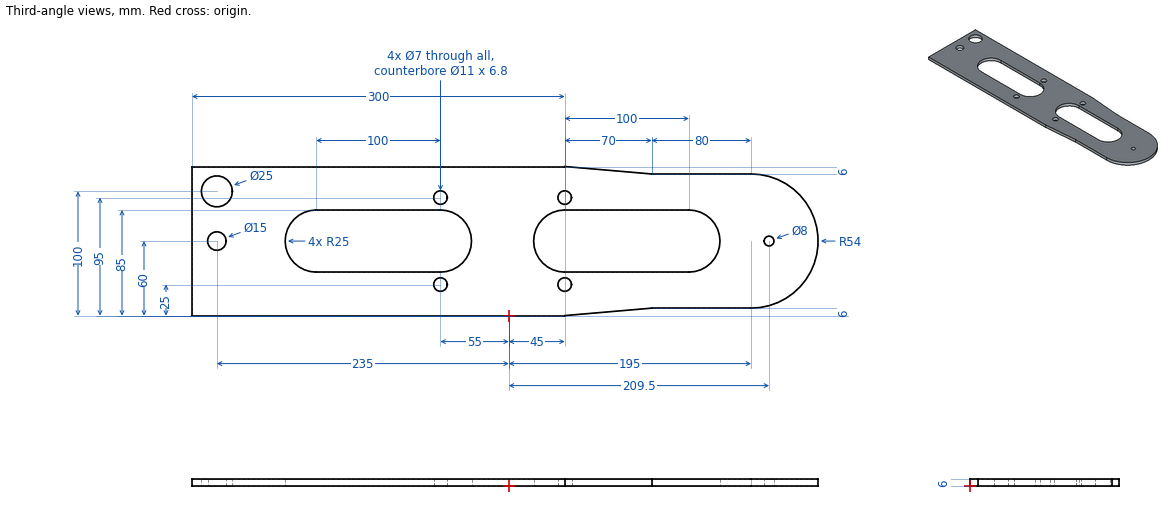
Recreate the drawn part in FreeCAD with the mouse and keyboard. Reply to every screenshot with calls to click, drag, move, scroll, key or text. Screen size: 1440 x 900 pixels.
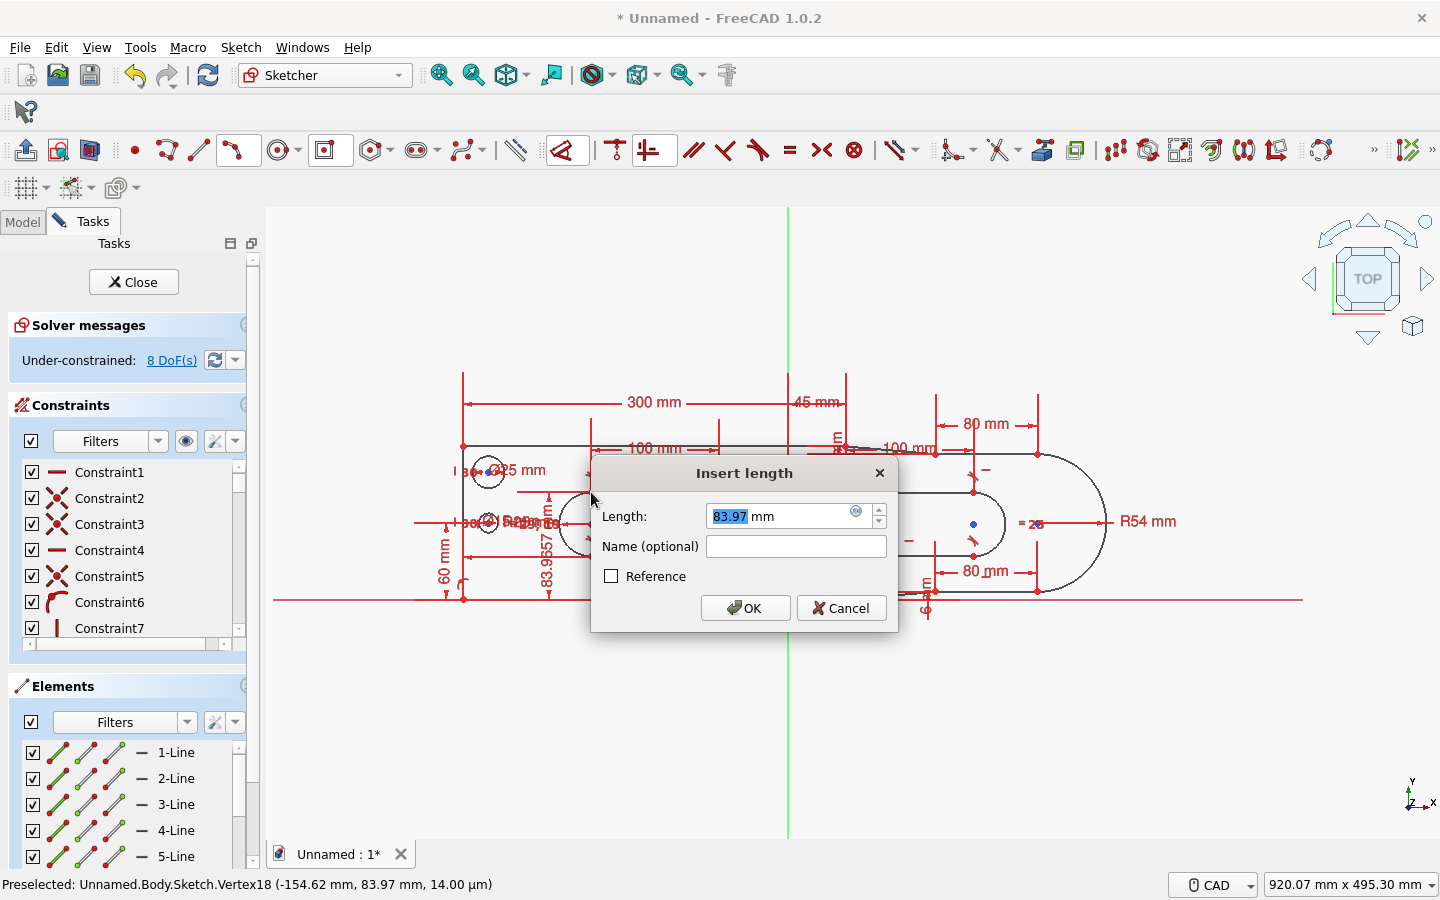
text(85)
key(Return)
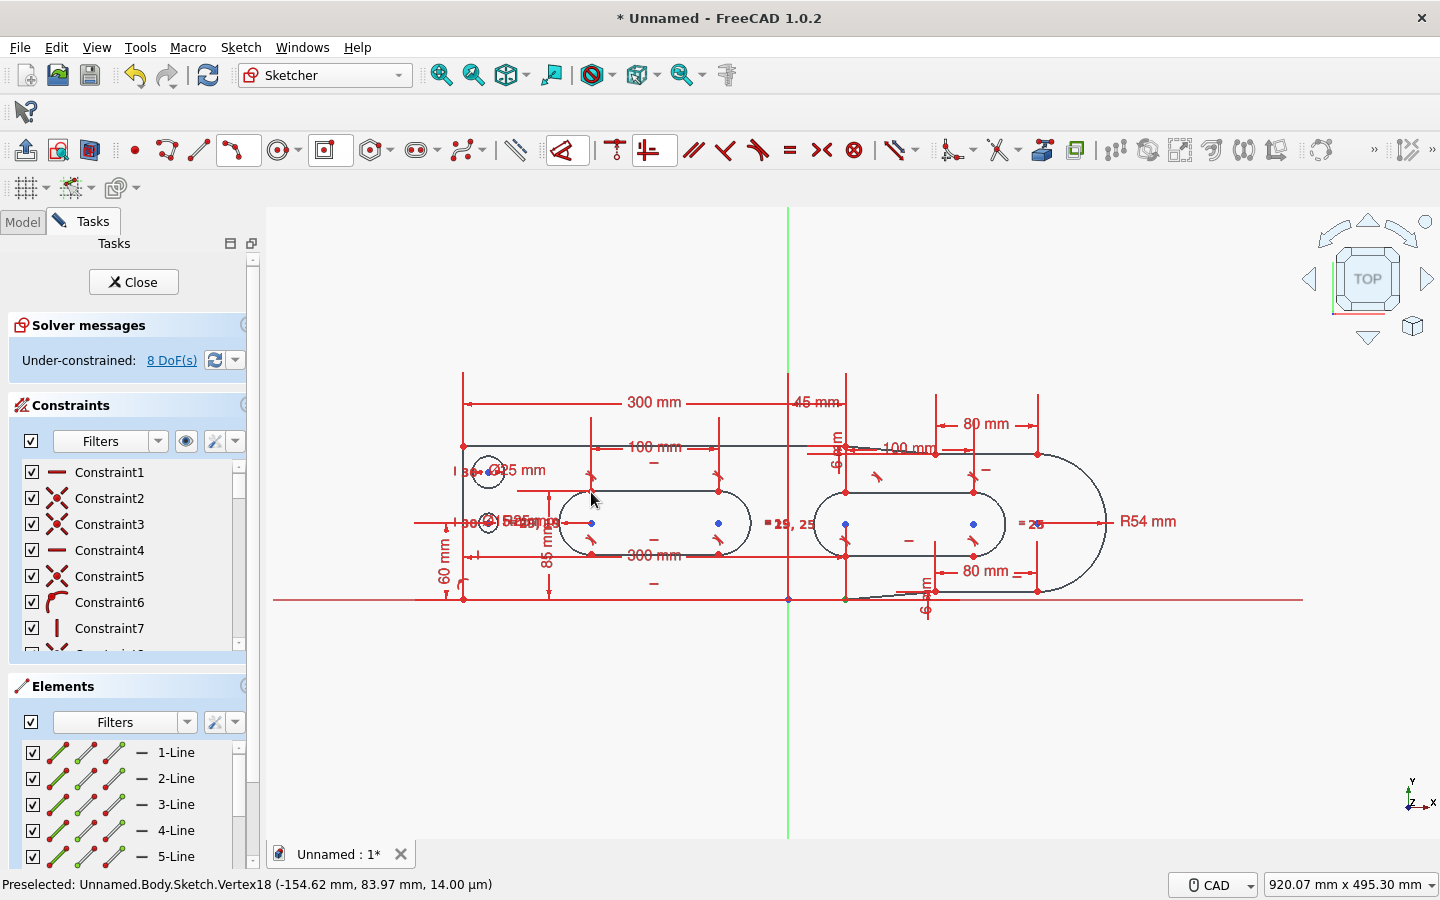
click(719, 555)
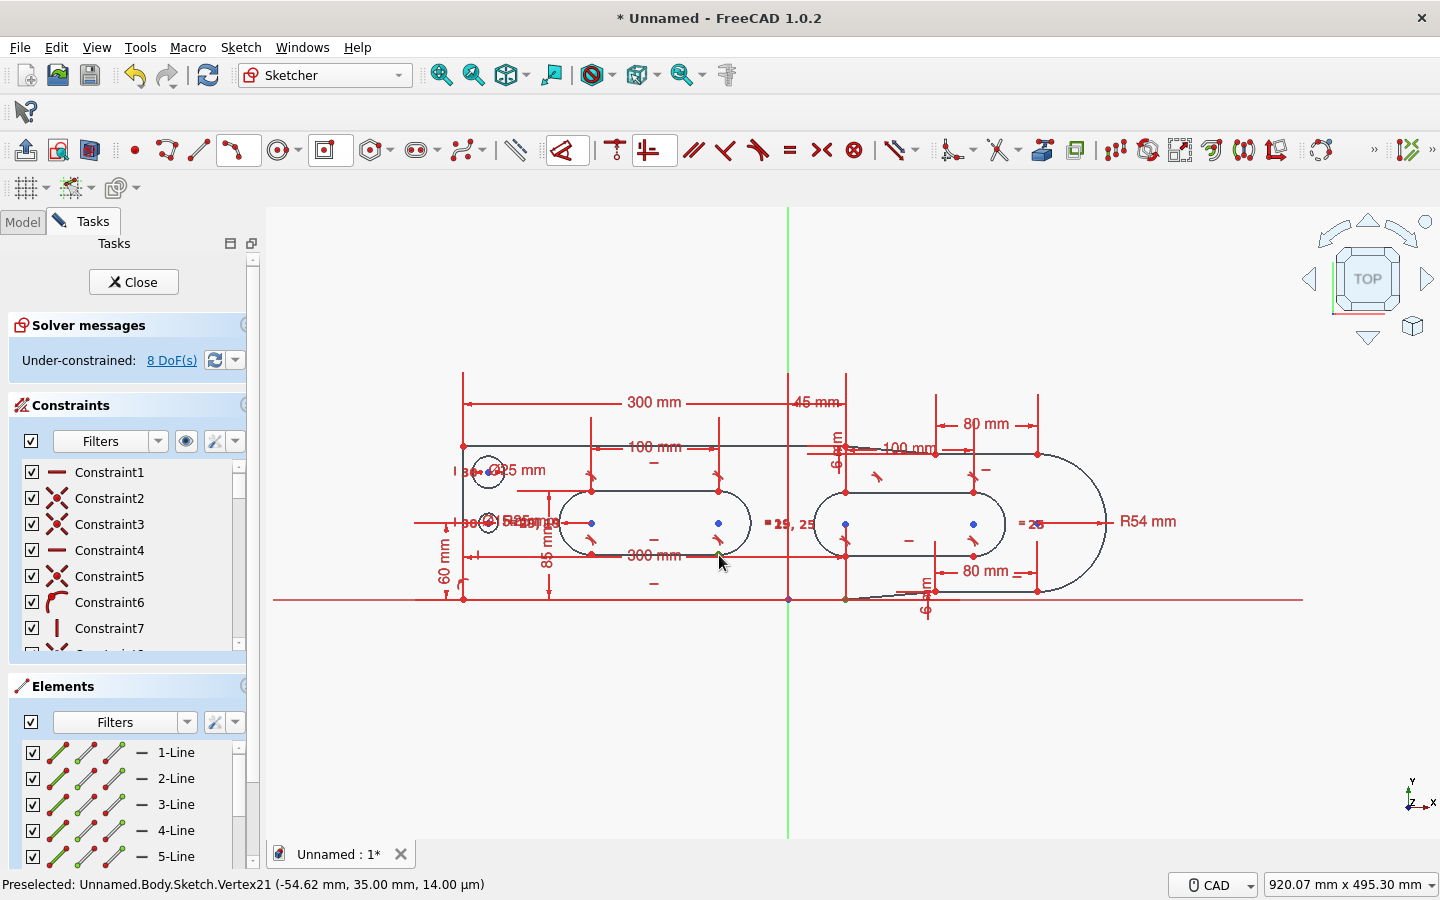
key(l)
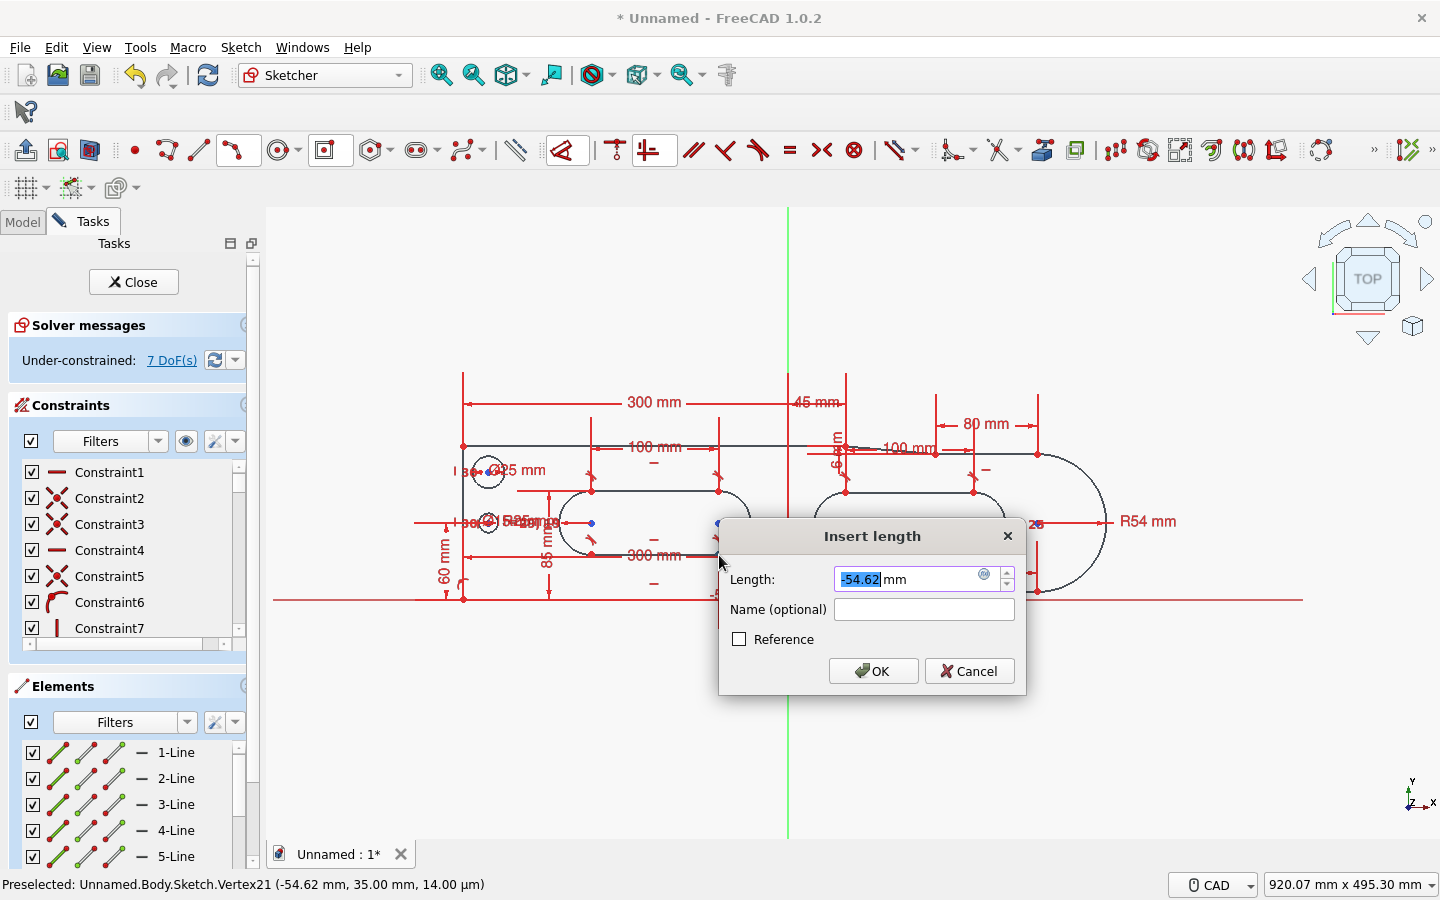
text(-55)
key(Return)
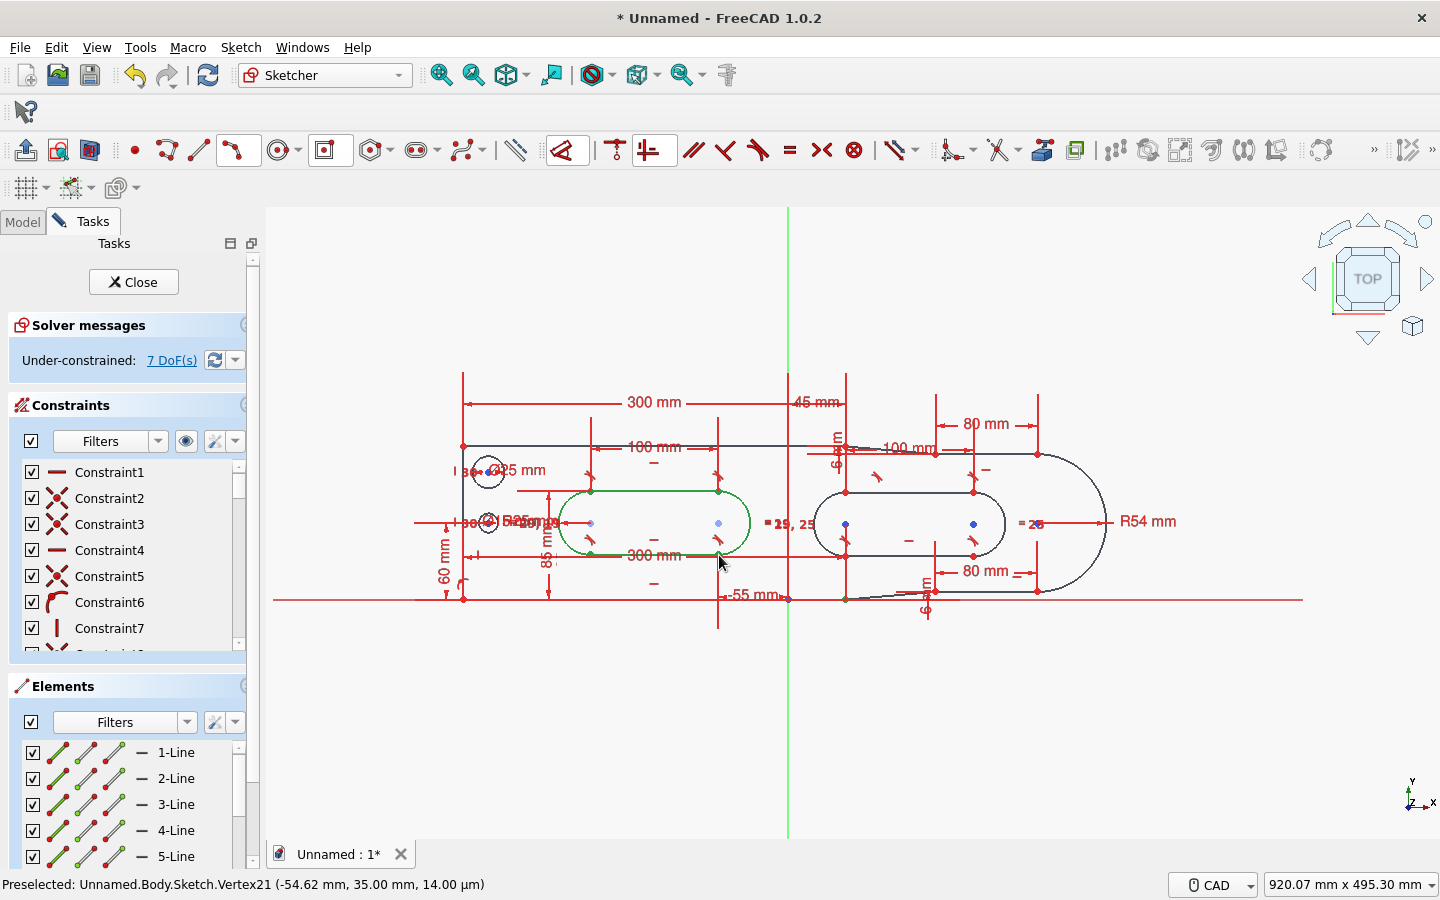
click(846, 493)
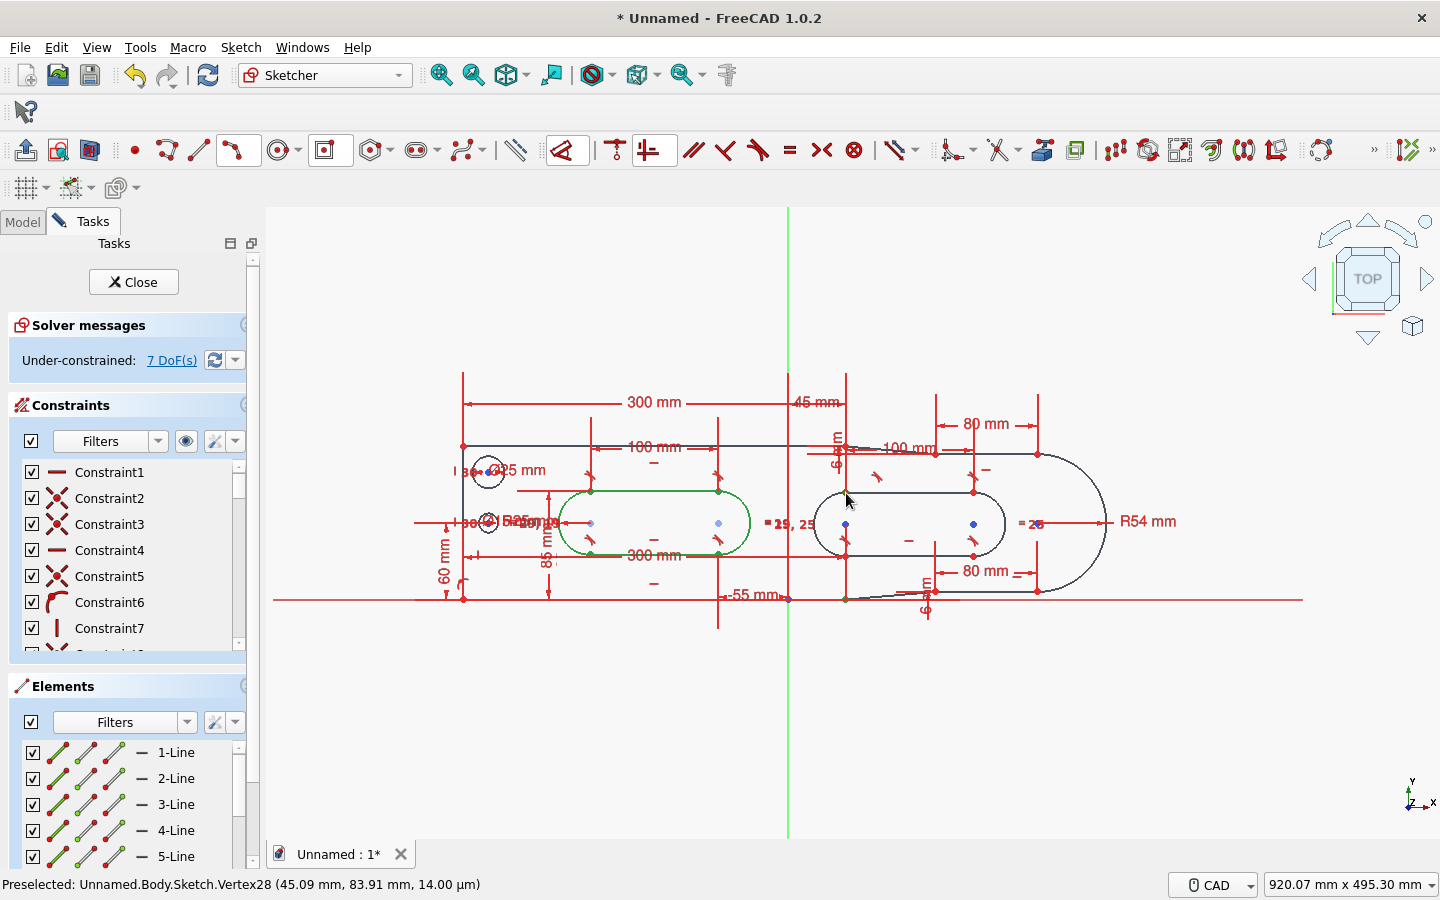
key(l)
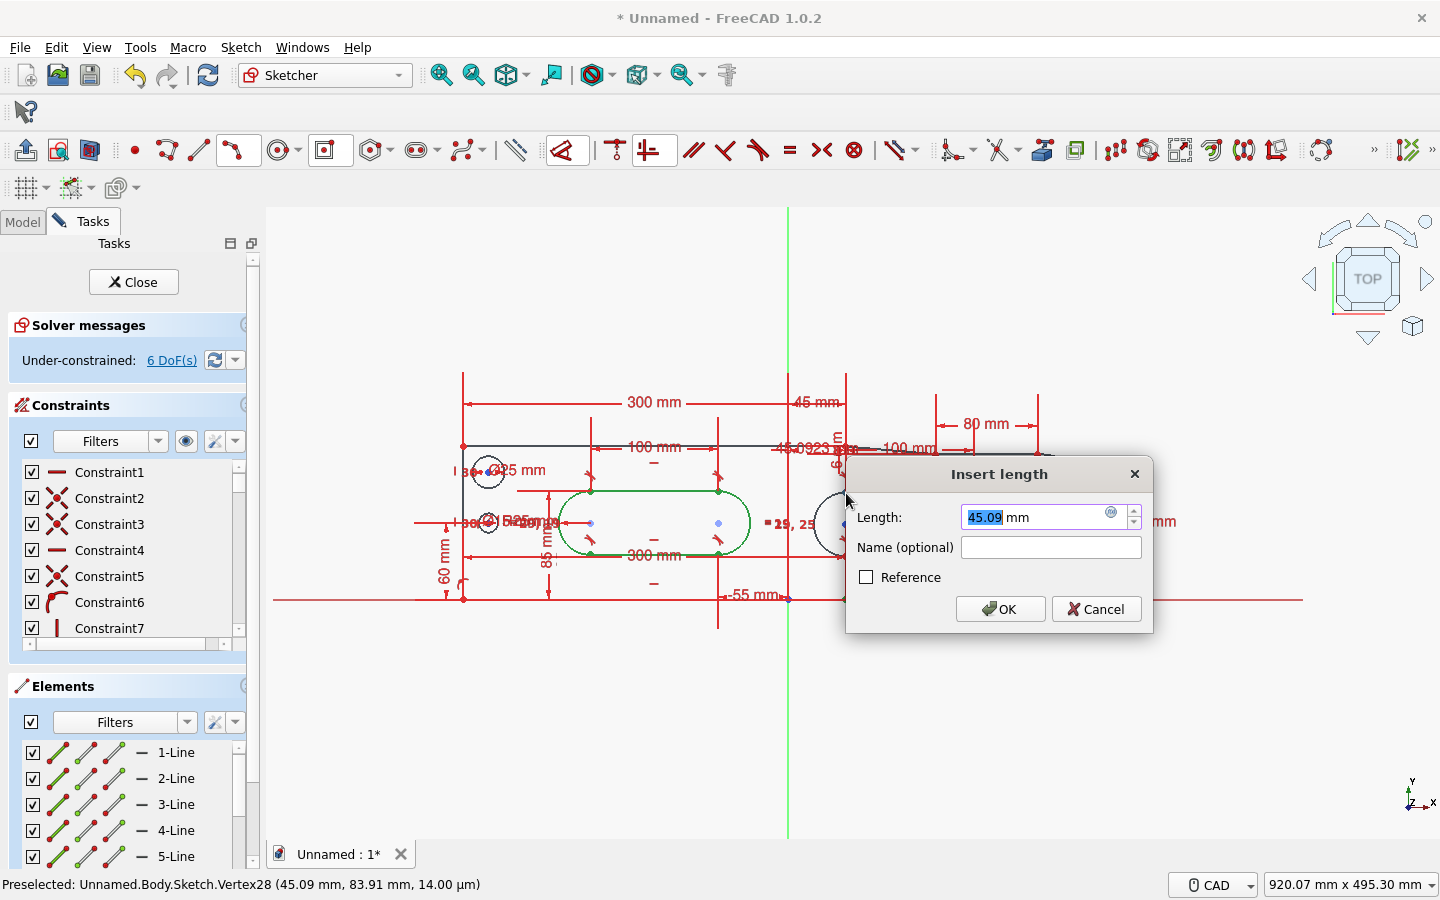
text(45)
key(Return)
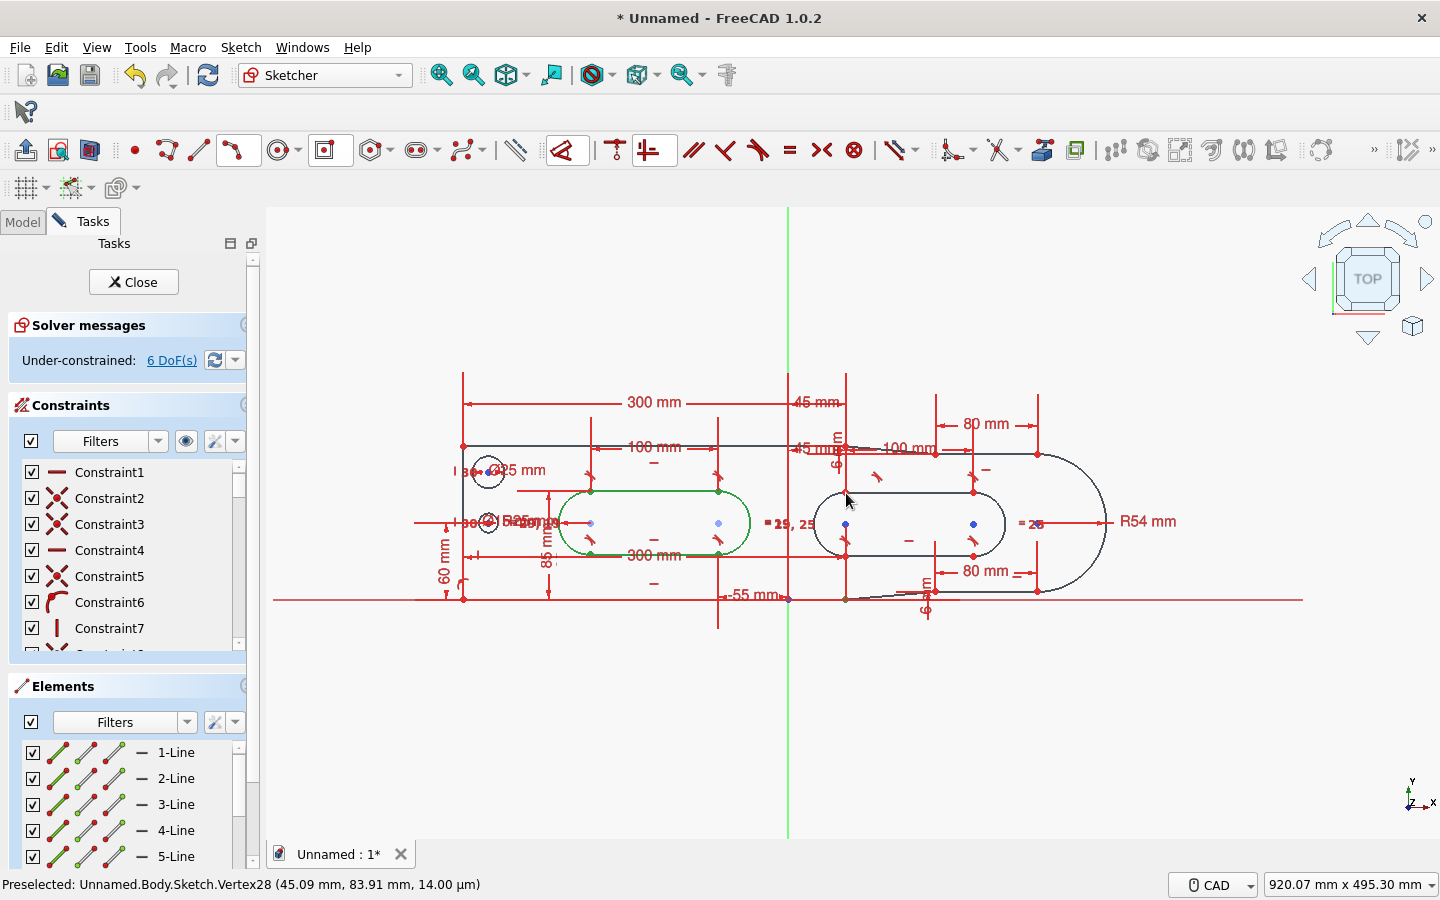
click(846, 493)